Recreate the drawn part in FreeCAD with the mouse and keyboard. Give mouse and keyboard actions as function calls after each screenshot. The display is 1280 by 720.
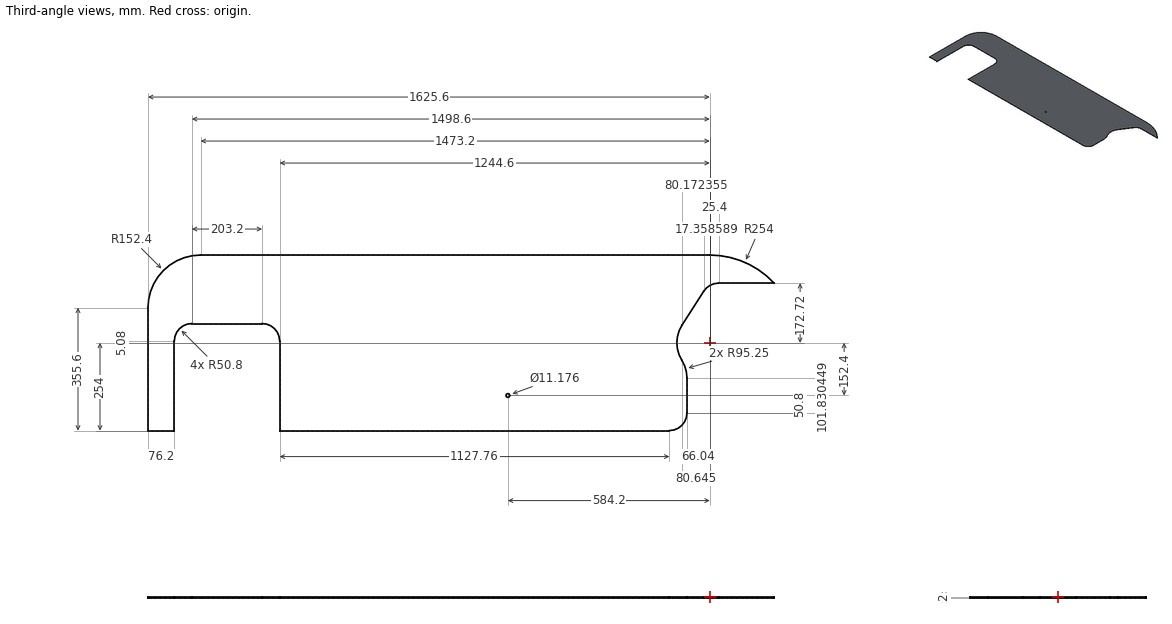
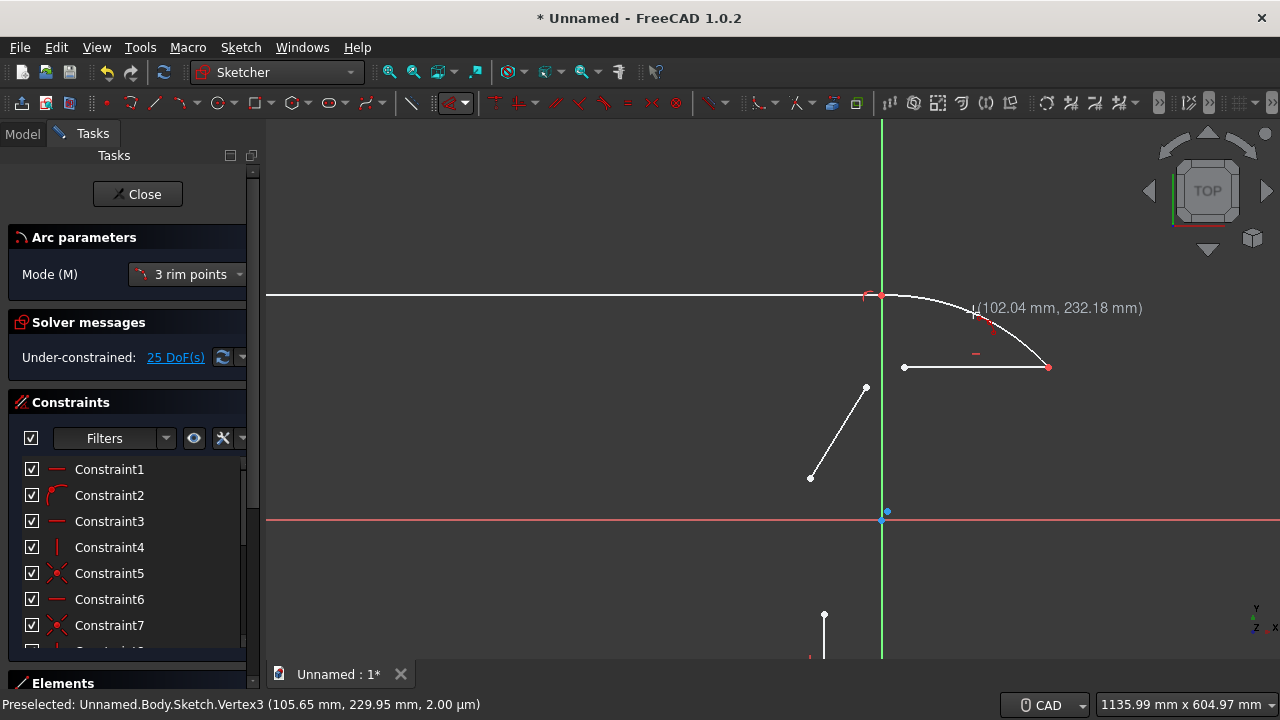
scroll(975, 313, down, 5)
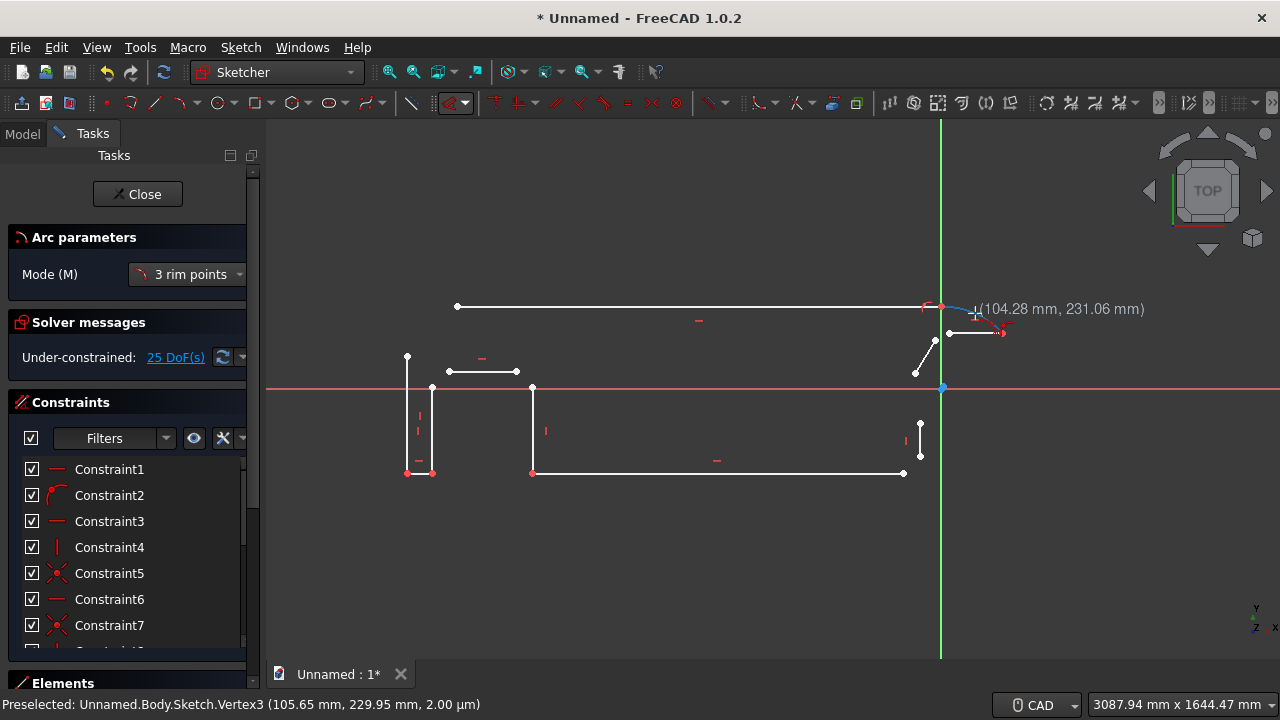
click(457, 307)
click(407, 357)
click(422, 321)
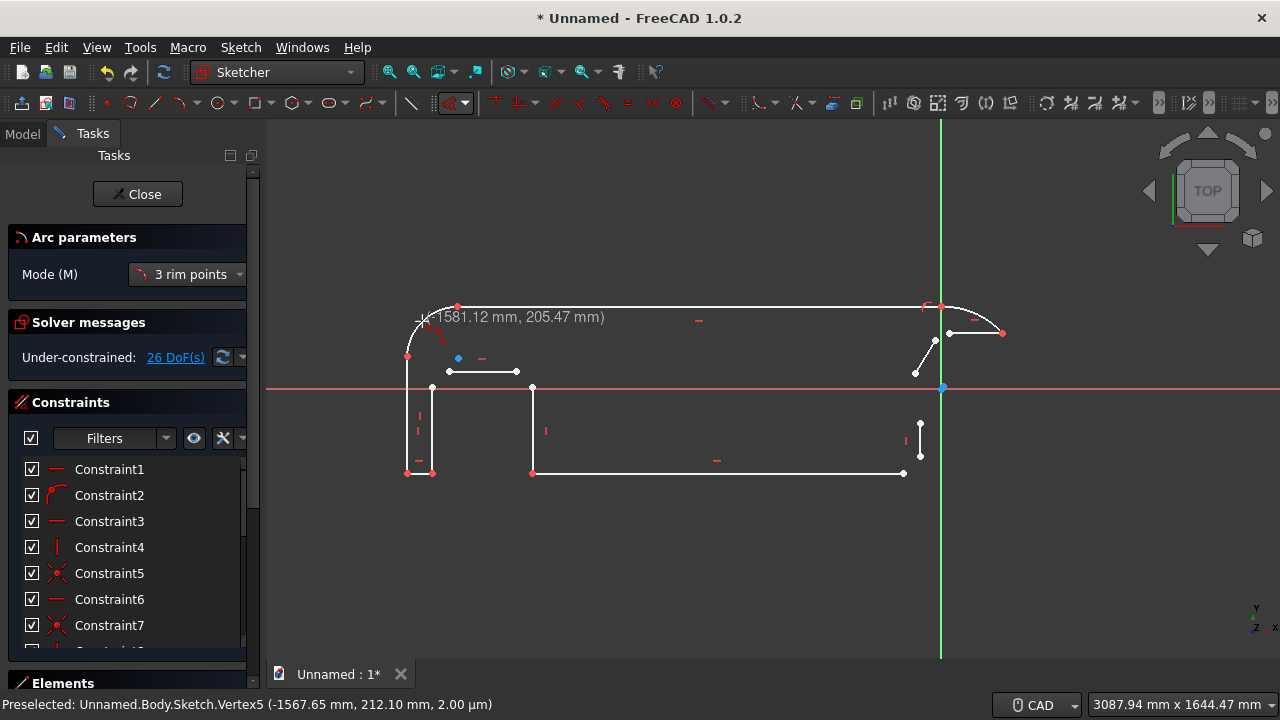
scroll(432, 388, up, 12)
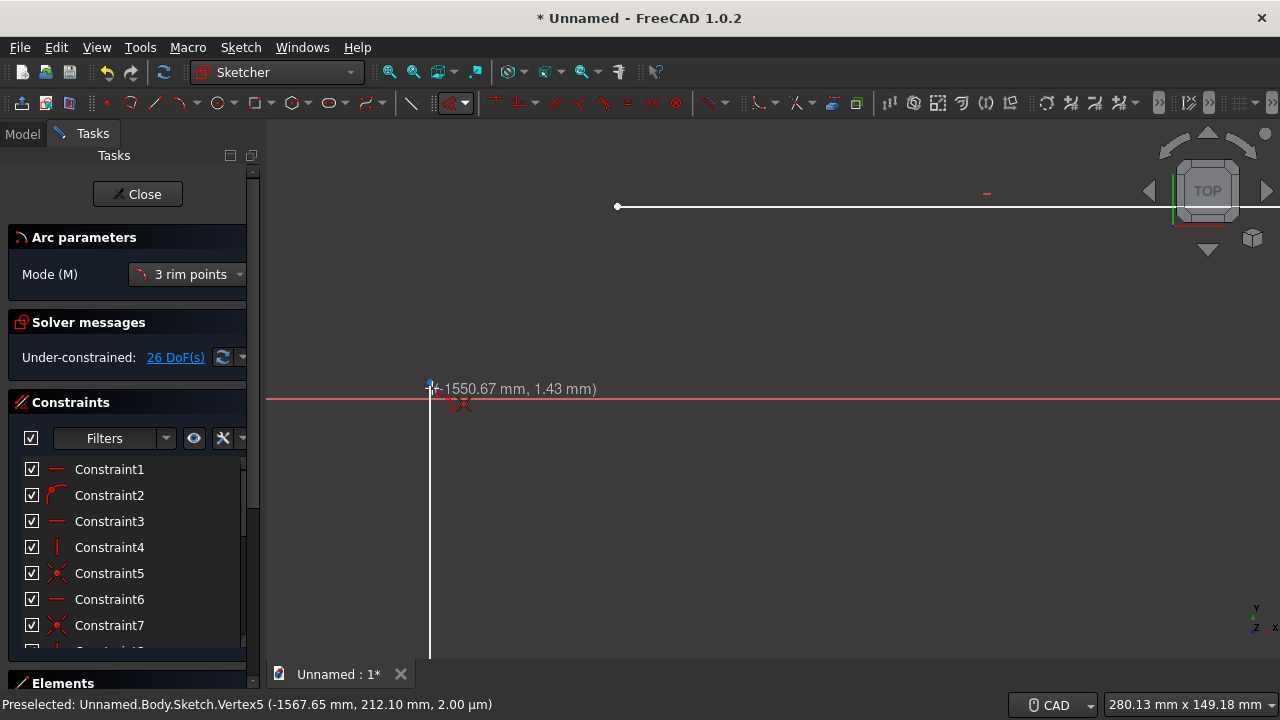
click(430, 382)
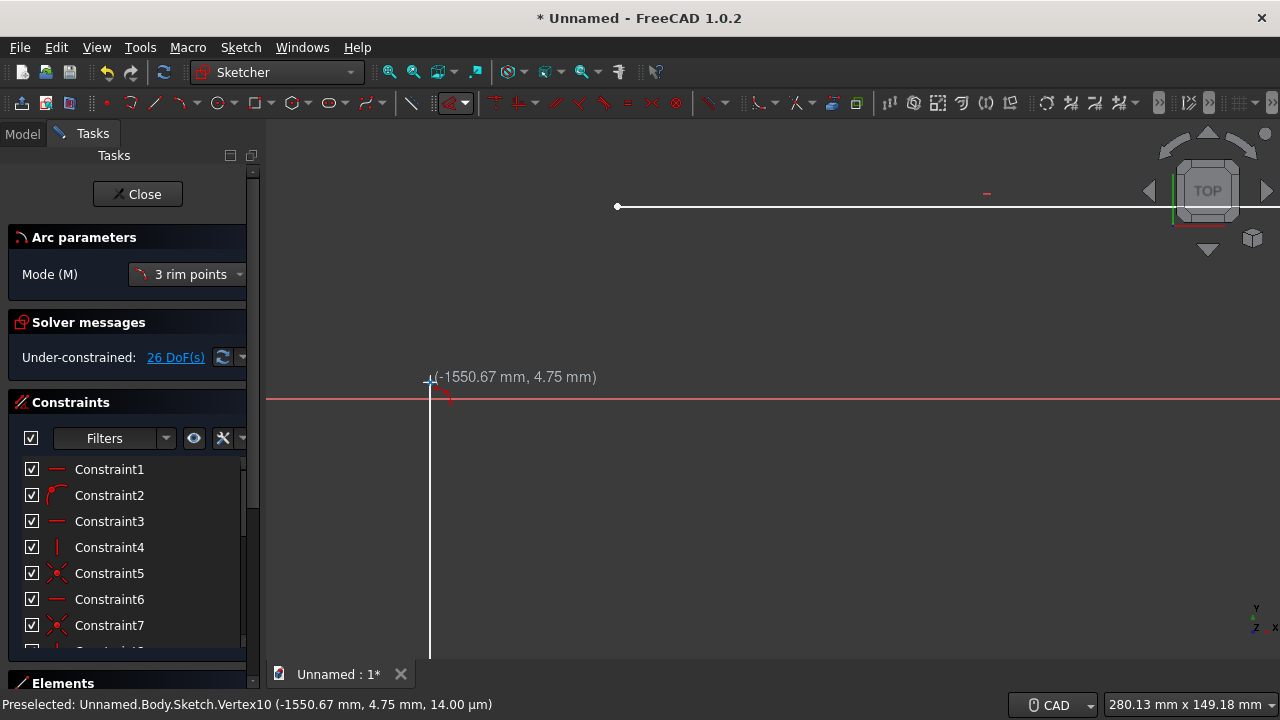
scroll(432, 388, down, 12)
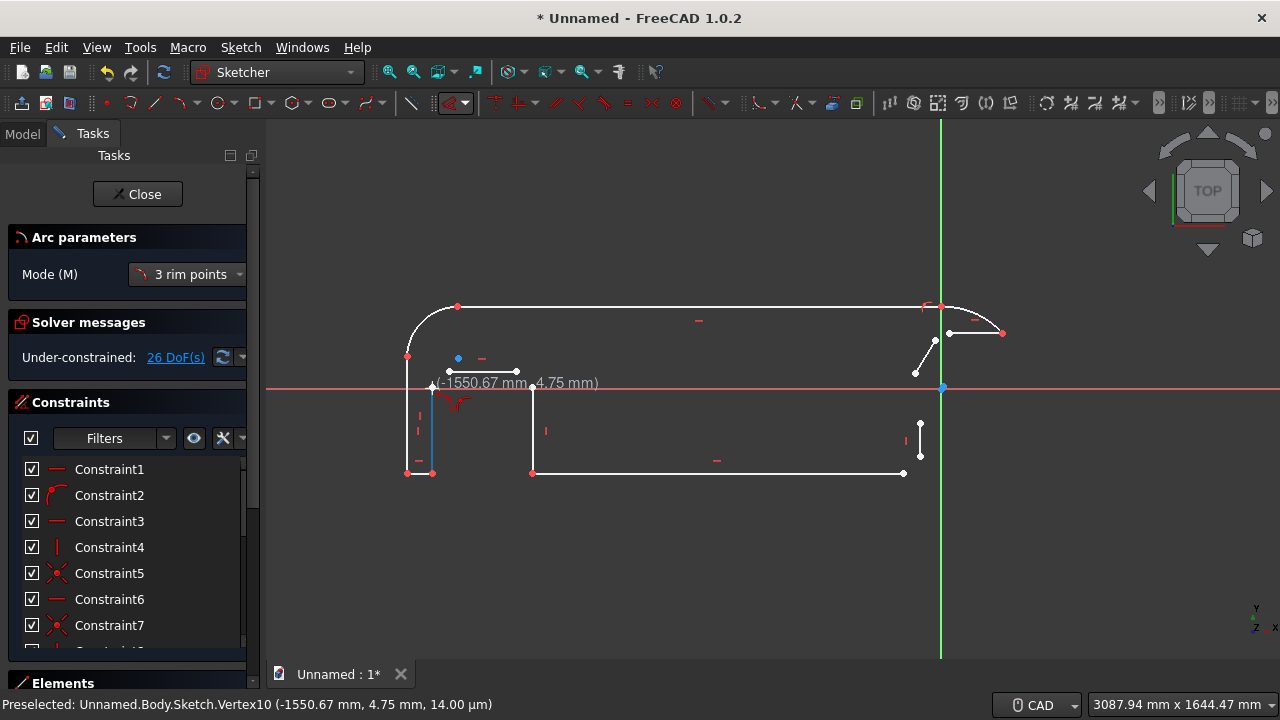
click(449, 372)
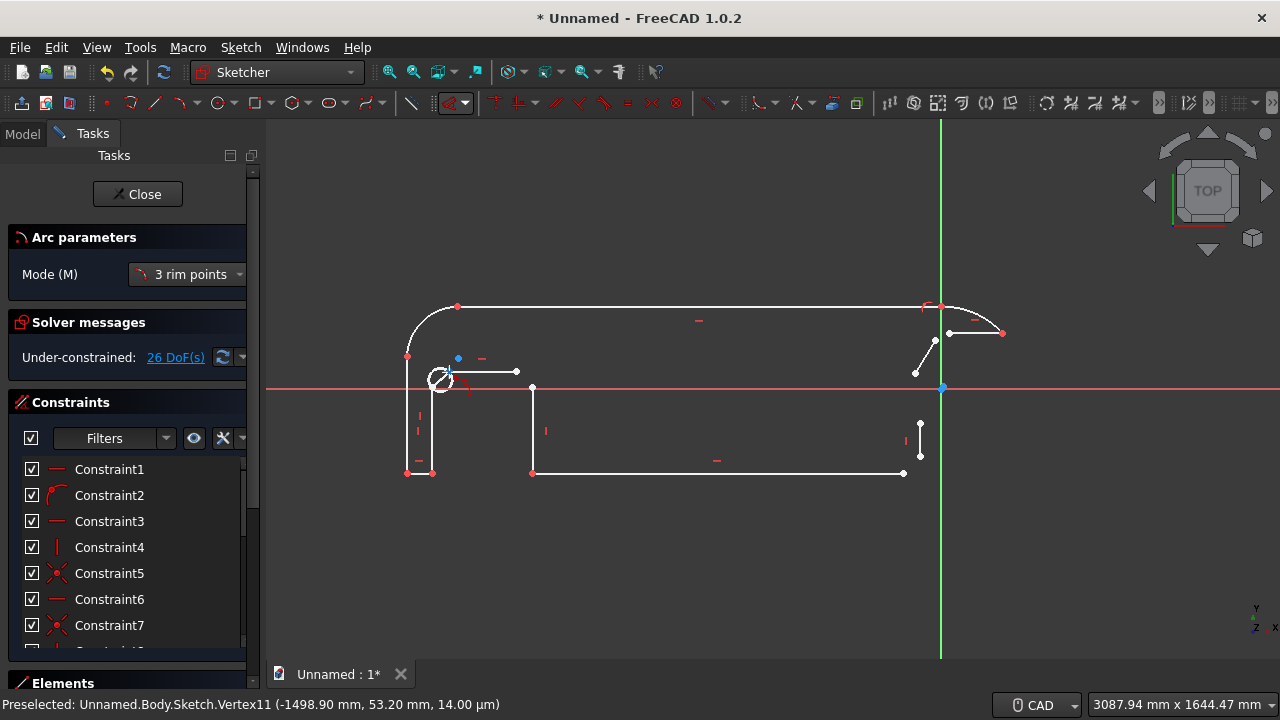
scroll(437, 376, up, 6)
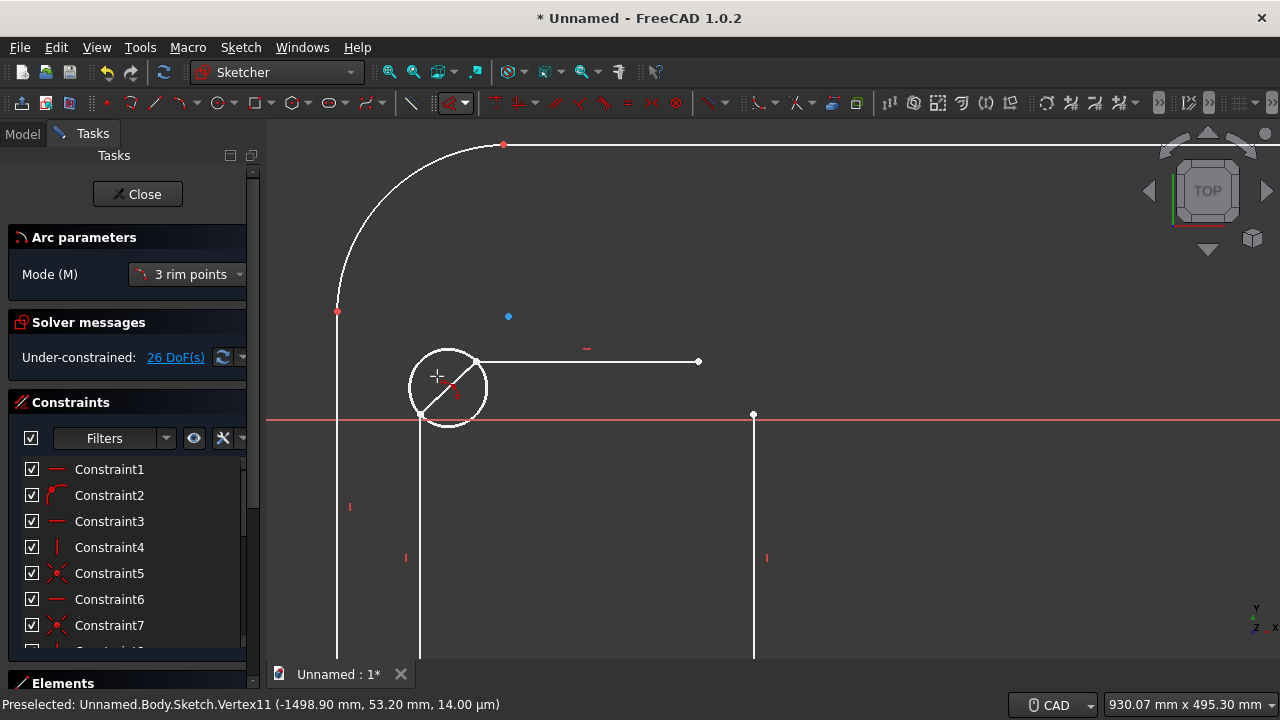
click(438, 375)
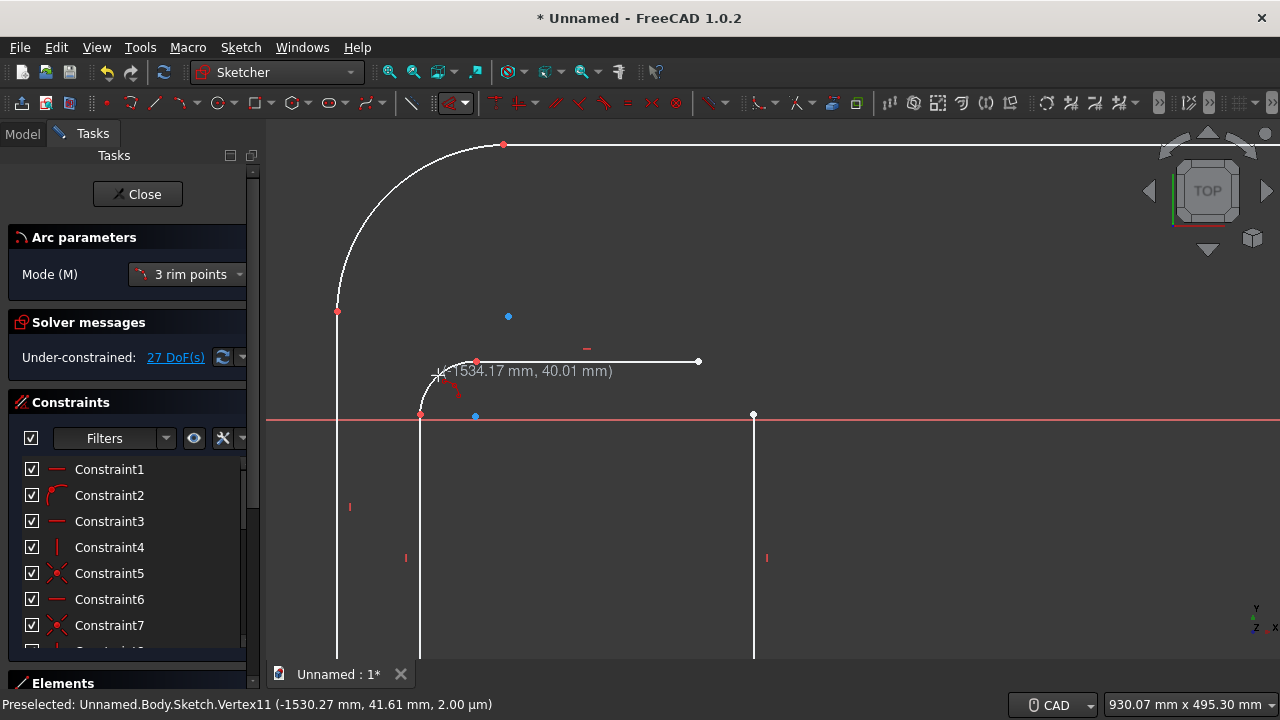
click(699, 362)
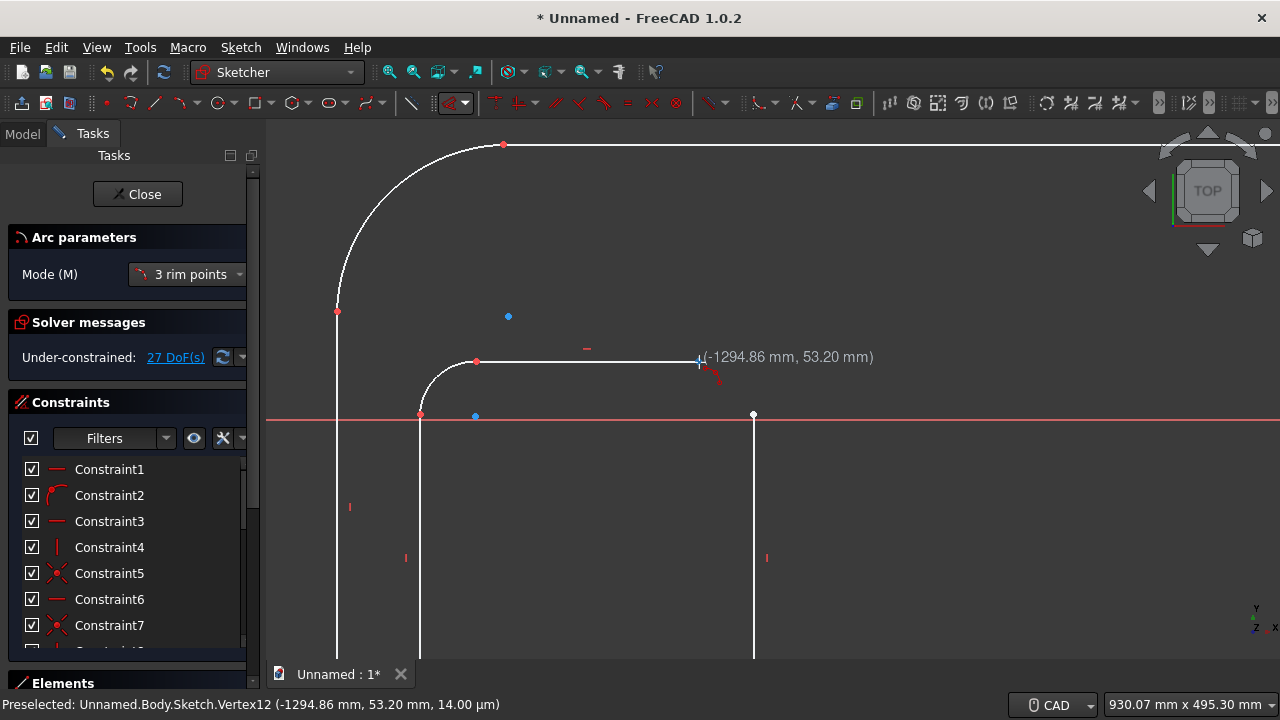
scroll(754, 414, up, 6)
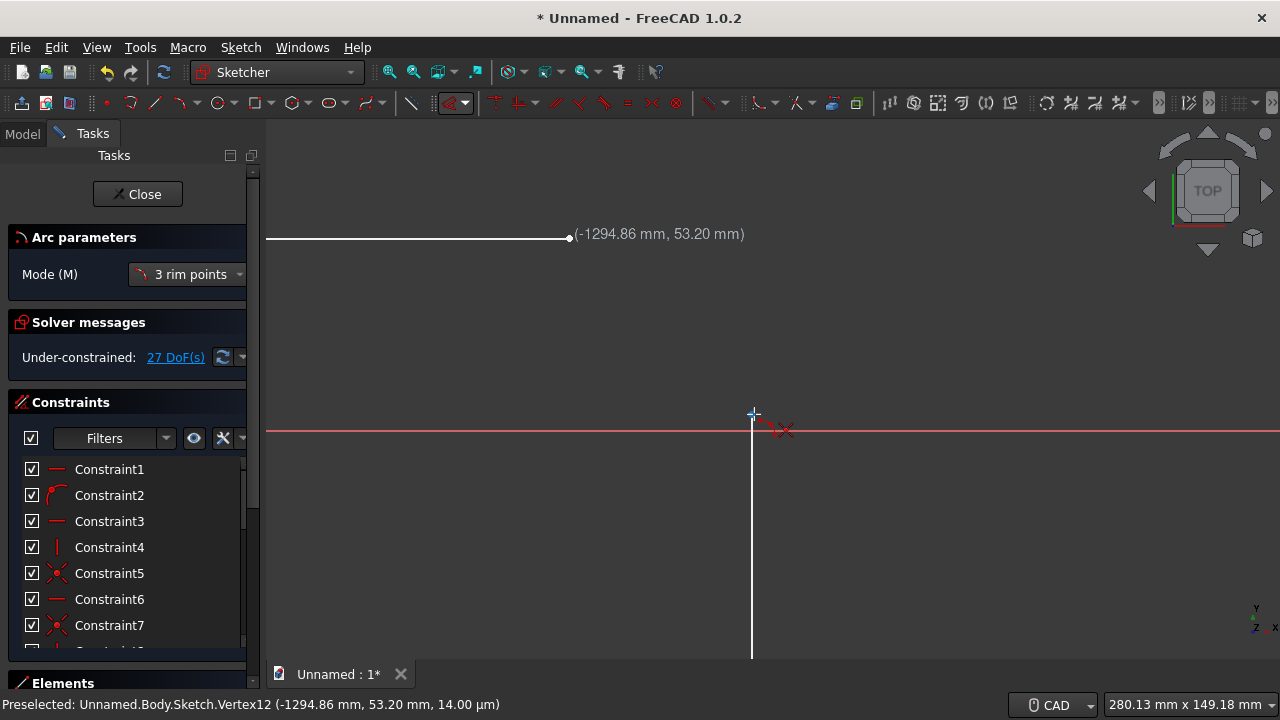
click(752, 414)